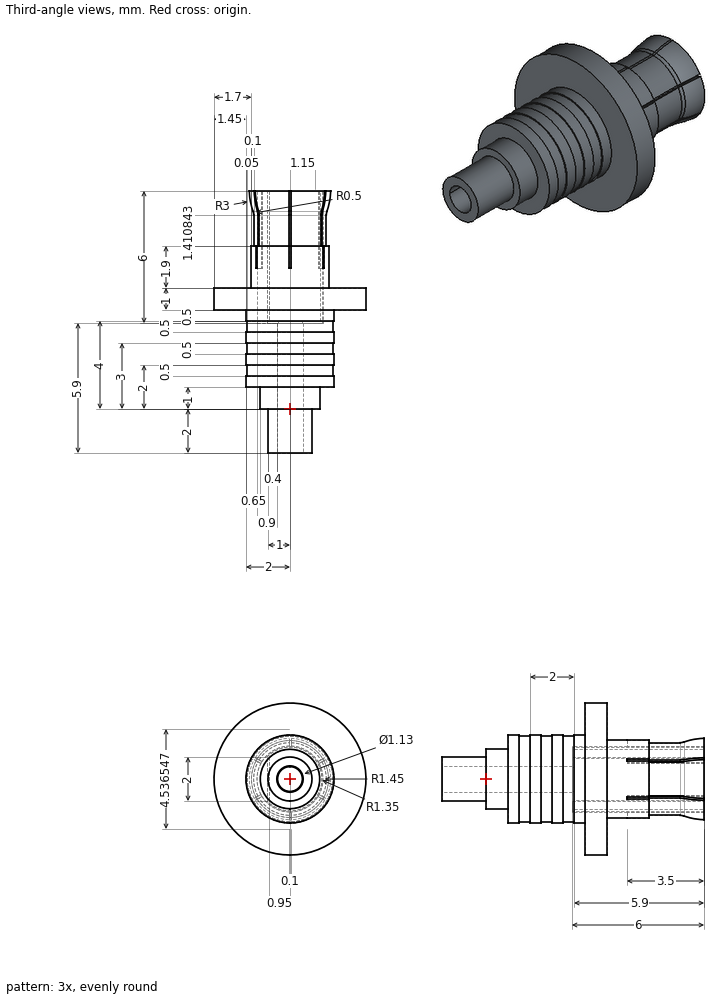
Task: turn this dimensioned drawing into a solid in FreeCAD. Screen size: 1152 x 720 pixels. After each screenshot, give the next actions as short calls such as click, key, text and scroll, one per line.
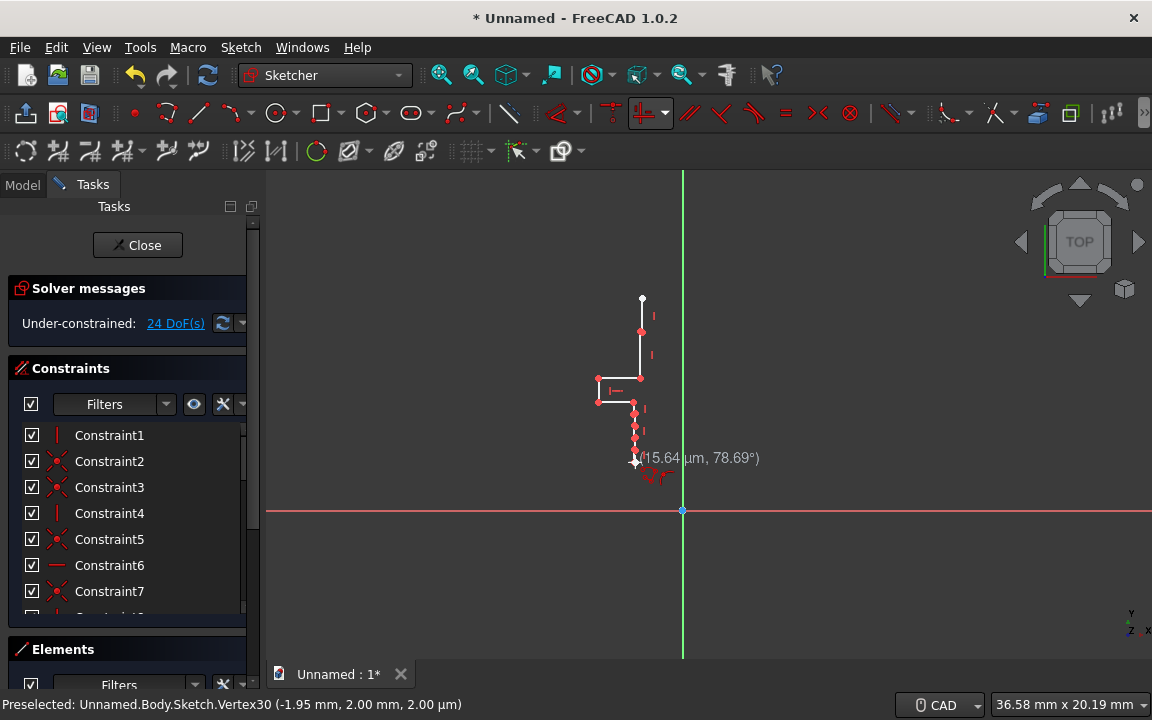
scroll(635, 474, up, 2)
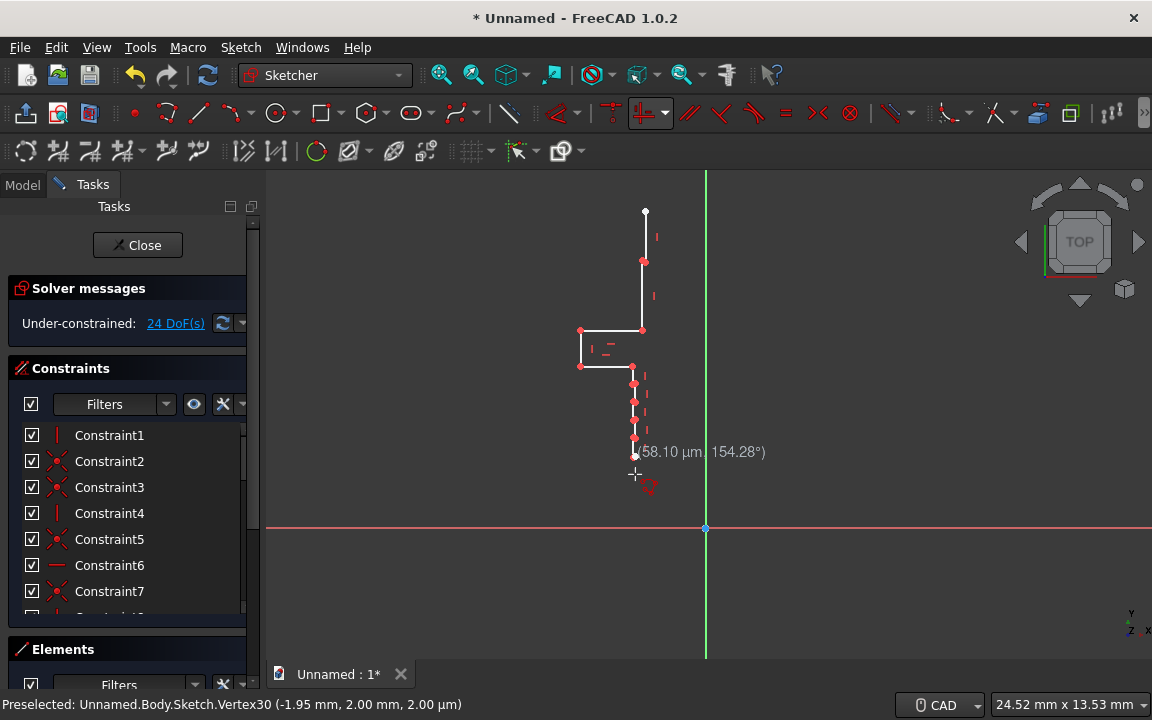
click(635, 474)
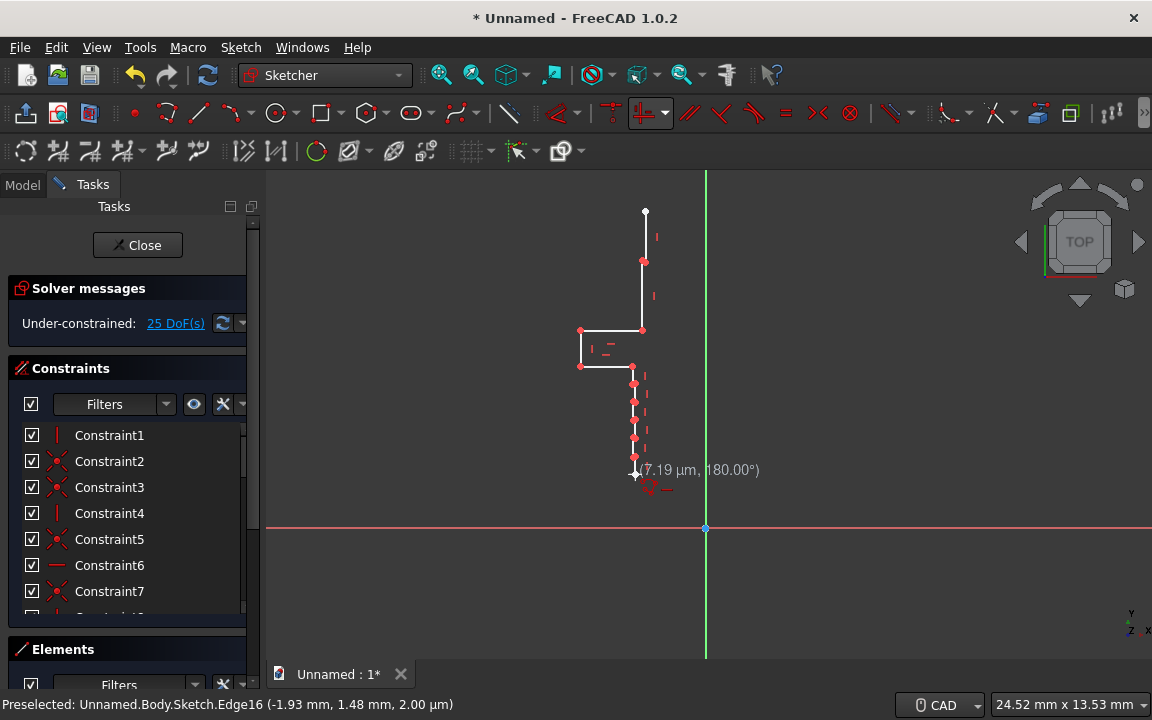
scroll(633, 474, up, 11)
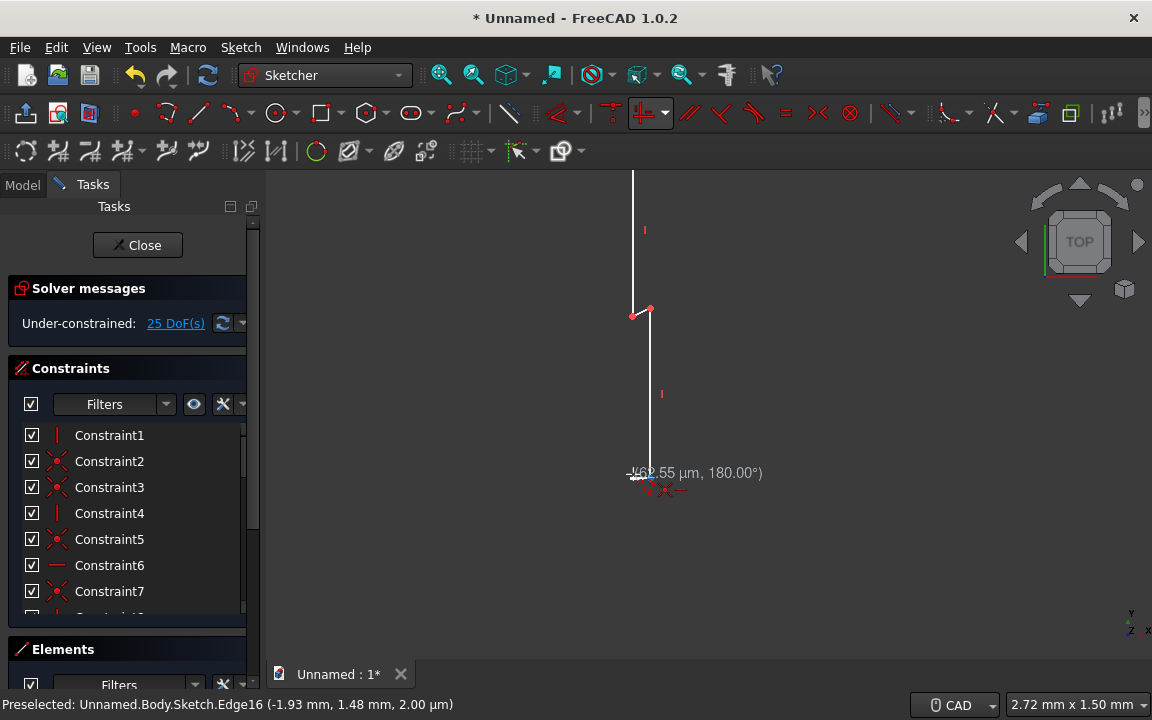
click(633, 469)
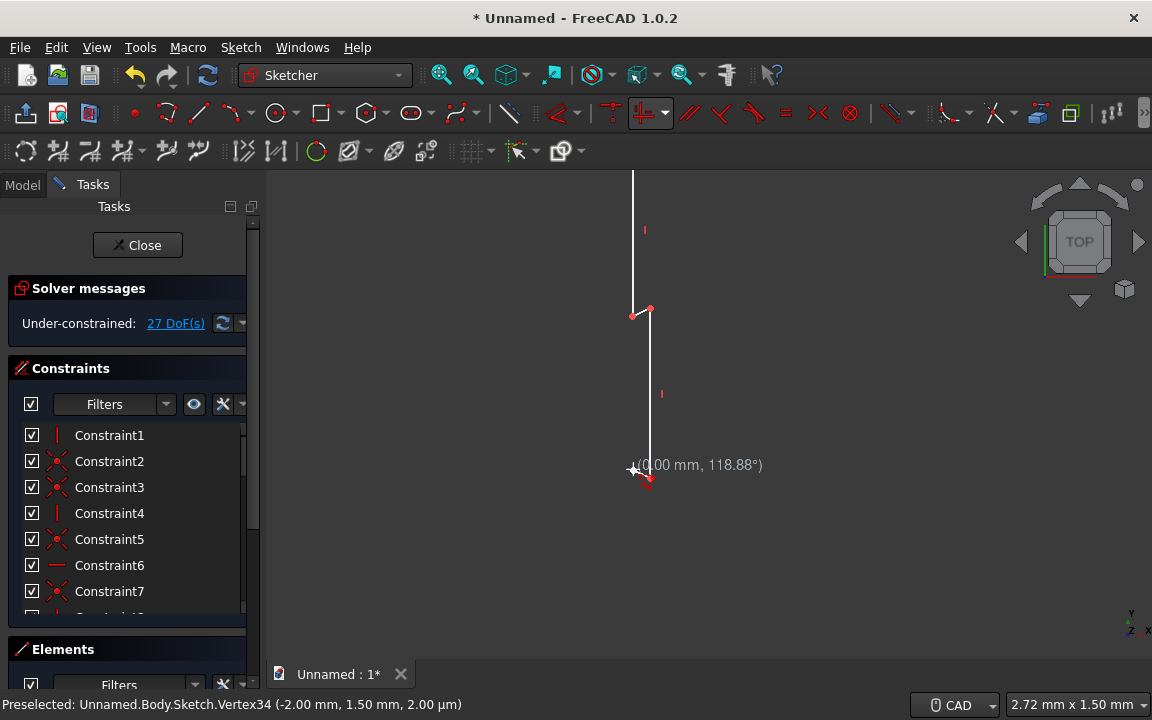
scroll(634, 474, down, 13)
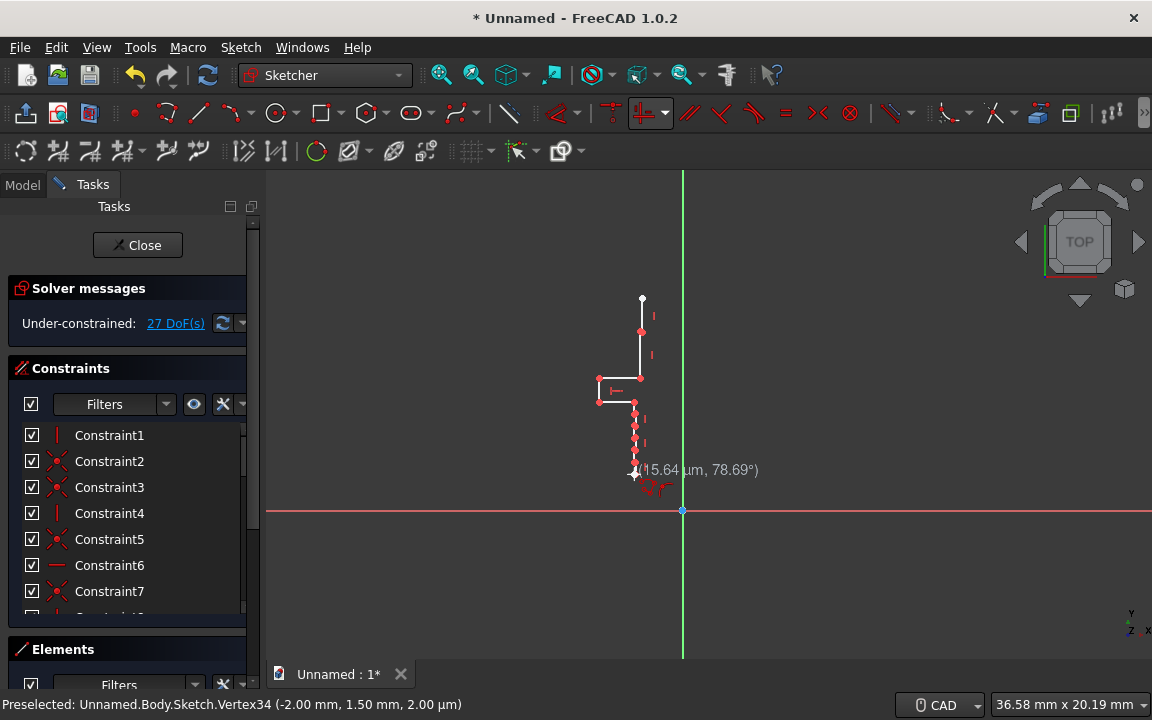
scroll(634, 486, up, 2)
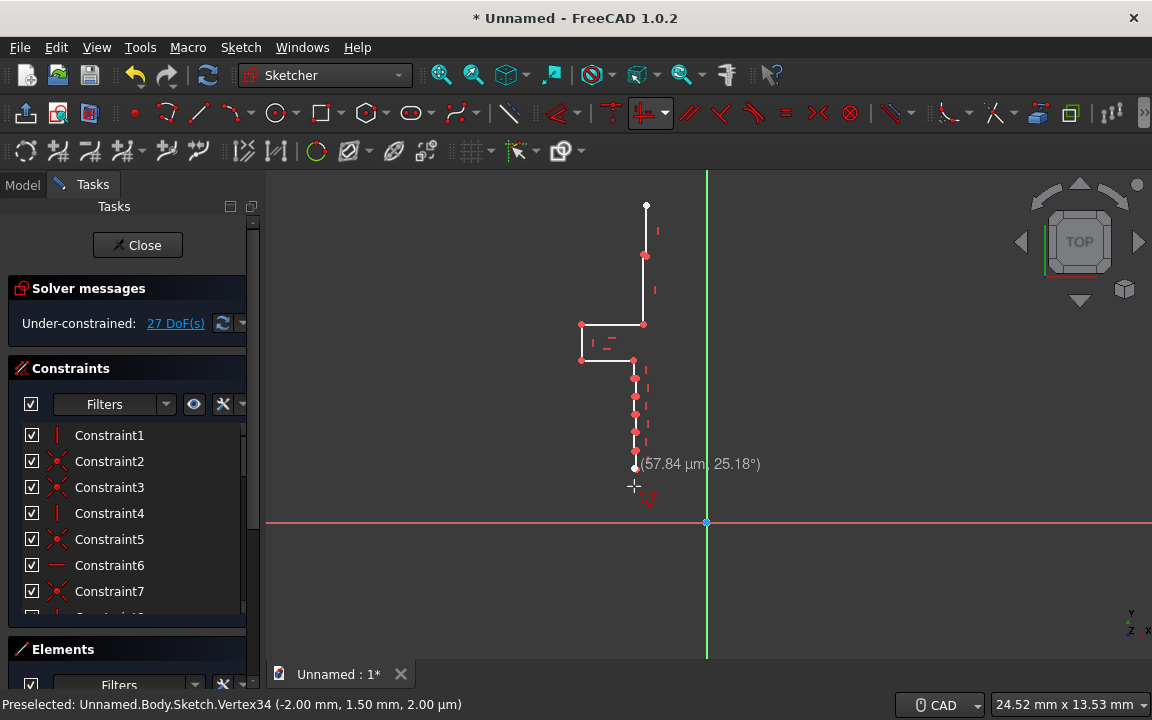
click(634, 486)
click(658, 486)
click(658, 523)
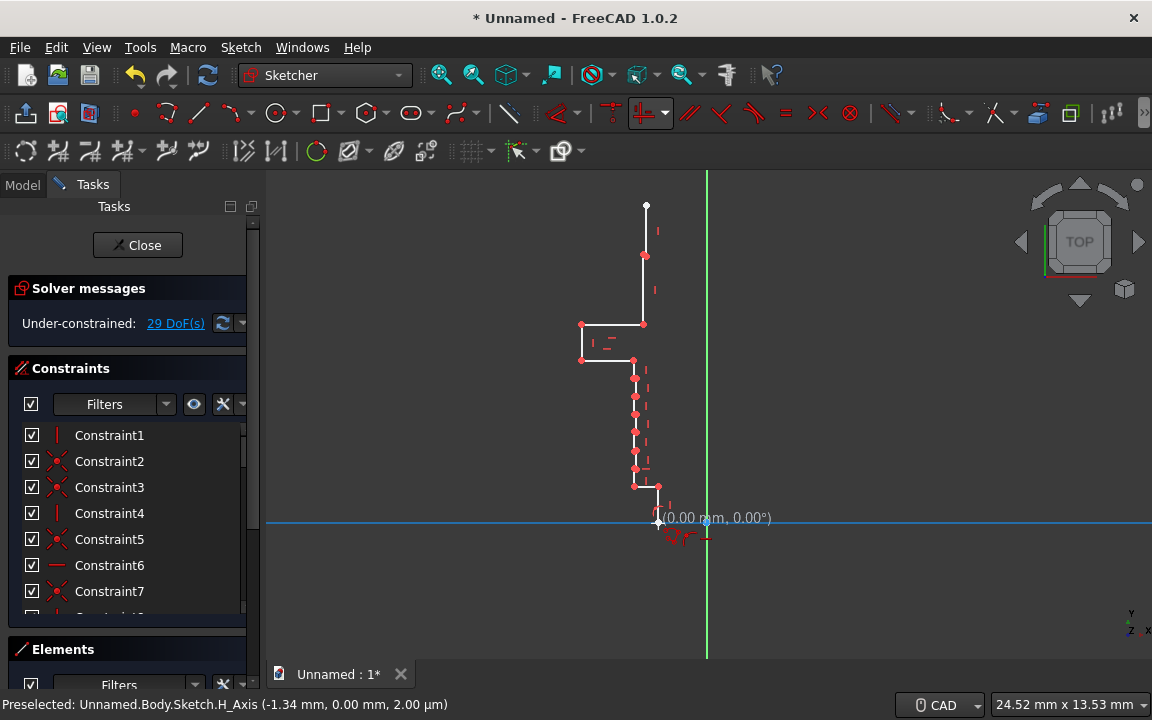
scroll(670, 523, up, 2)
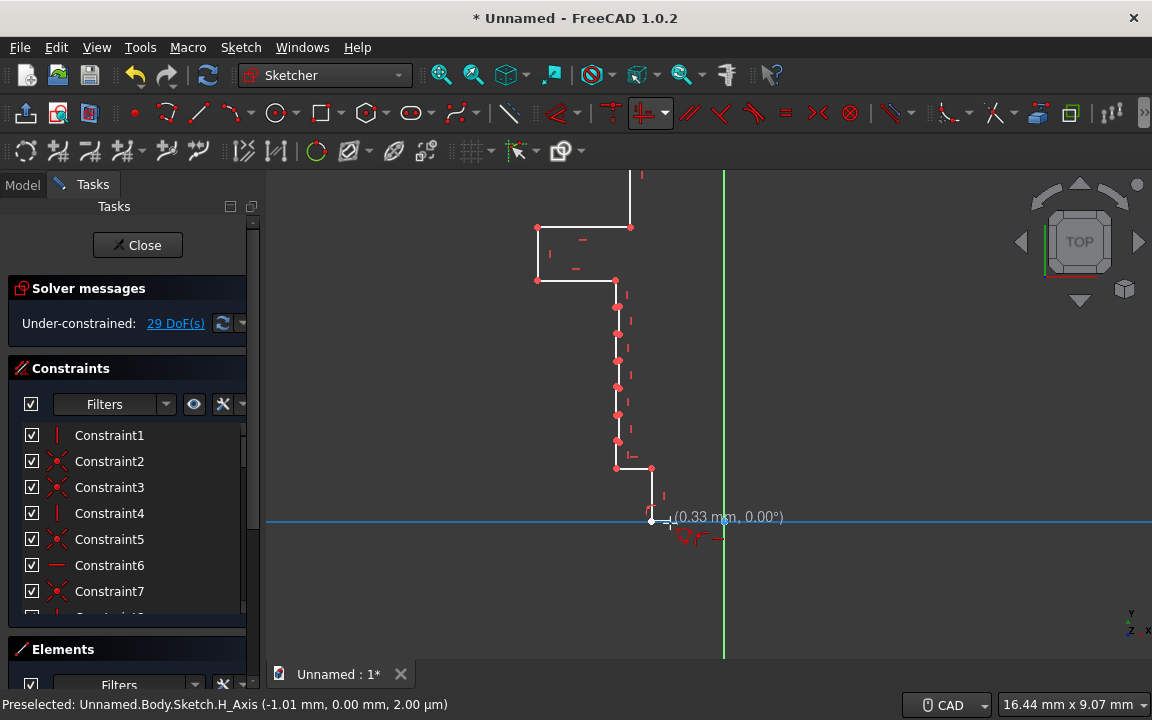
click(670, 513)
click(670, 630)
click(692, 630)
click(692, 312)
click(643, 312)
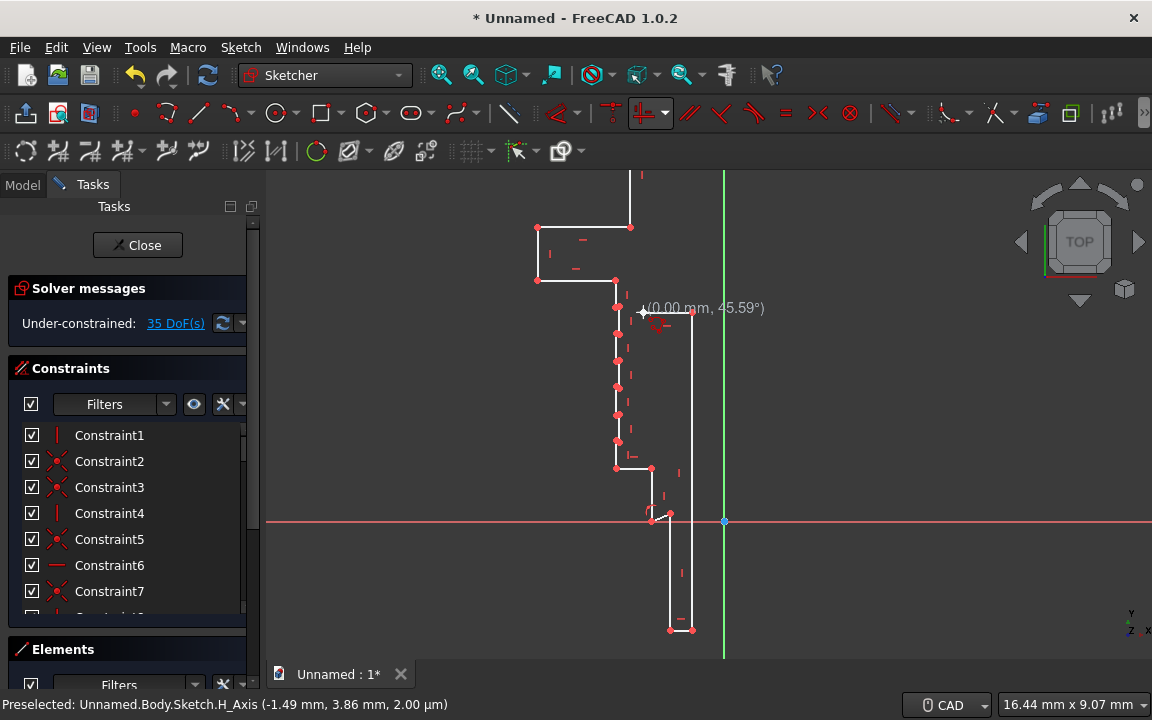
scroll(648, 501, down, 4)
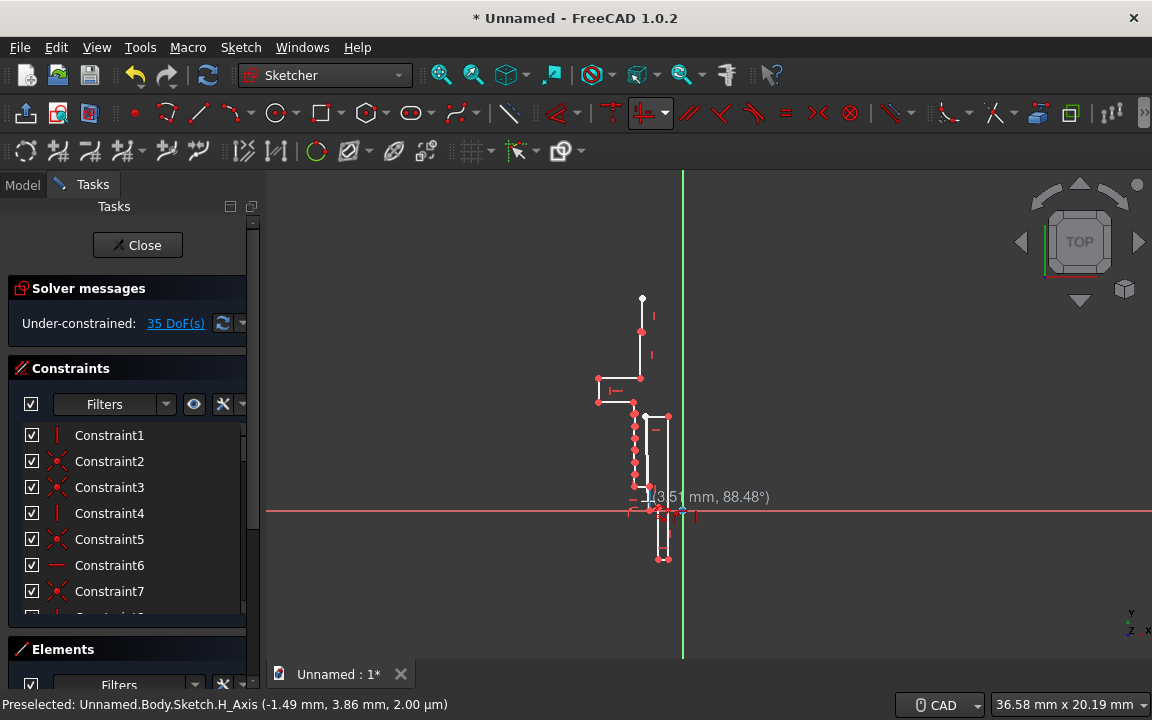
click(646, 271)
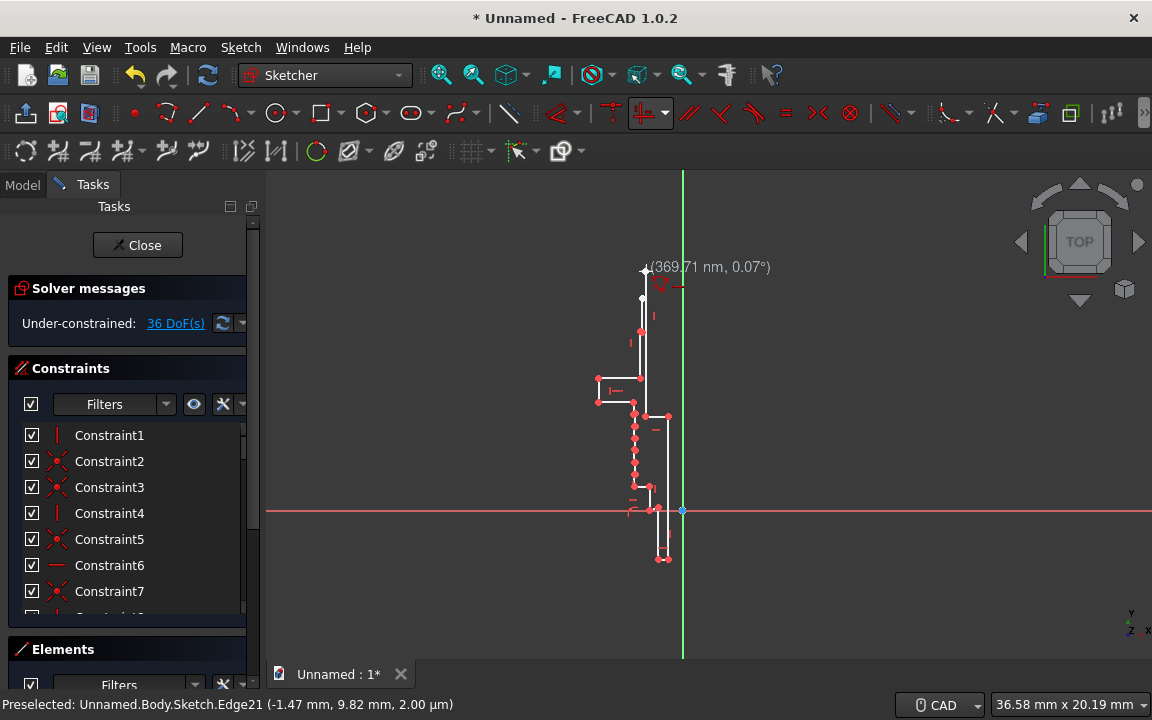
scroll(638, 271, up, 4)